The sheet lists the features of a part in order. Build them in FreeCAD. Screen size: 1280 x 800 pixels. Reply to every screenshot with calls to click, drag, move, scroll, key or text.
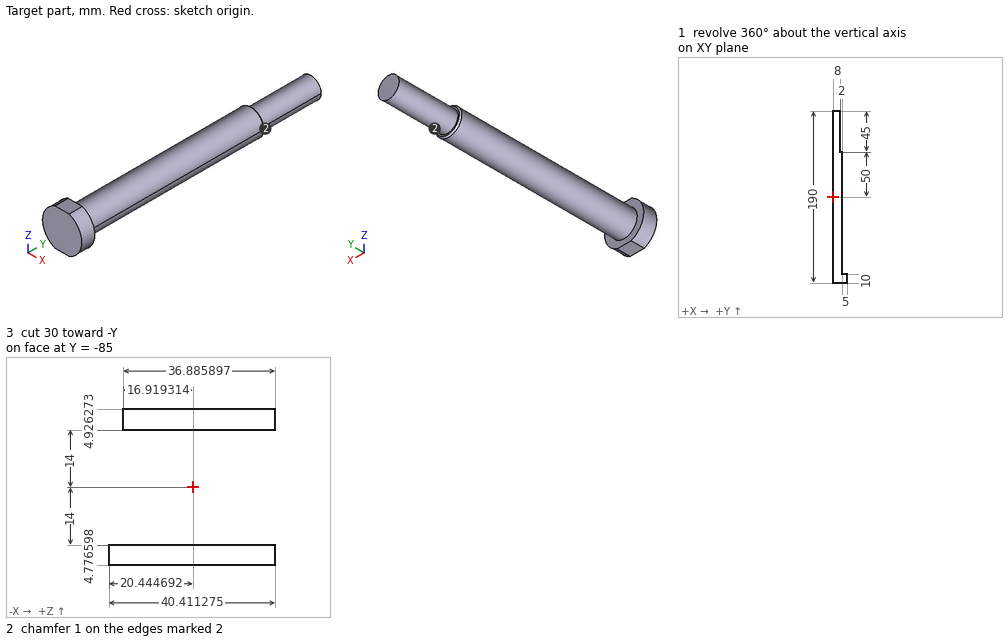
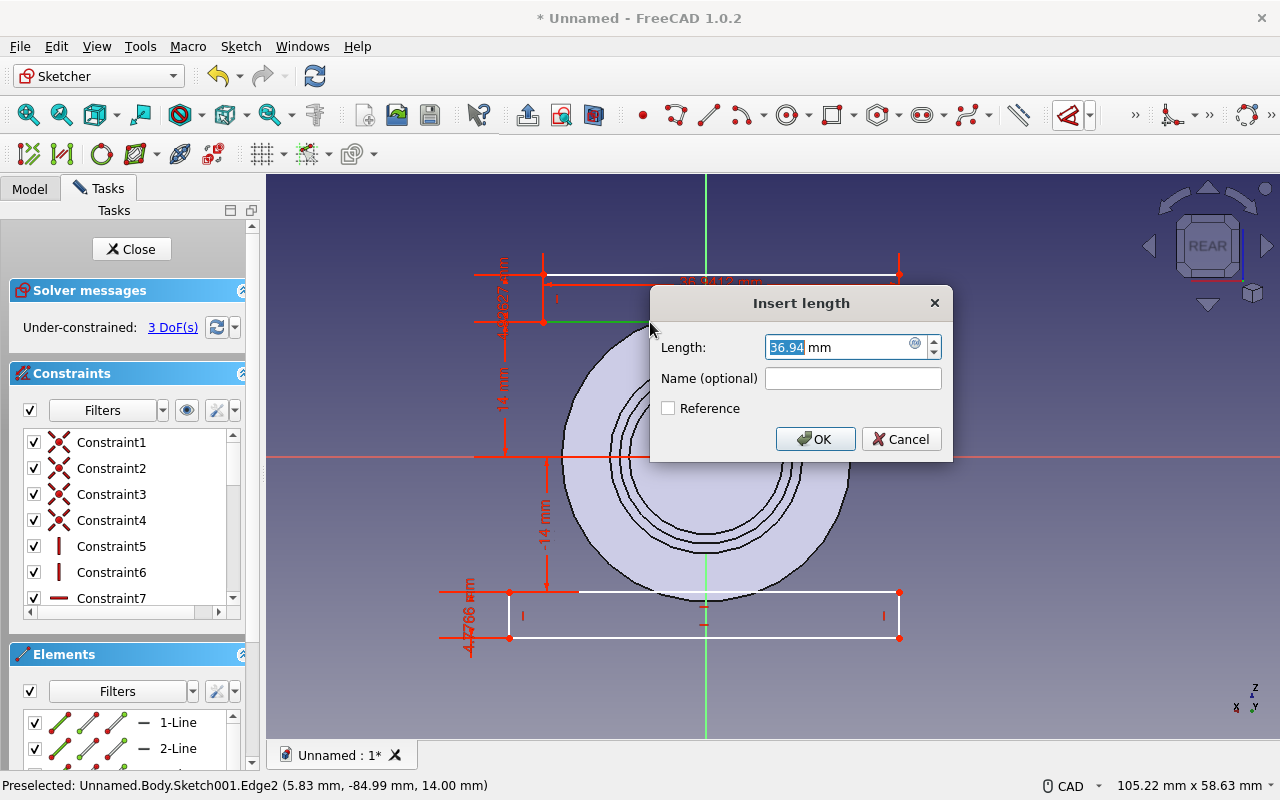
text(36.885897)
key(Return)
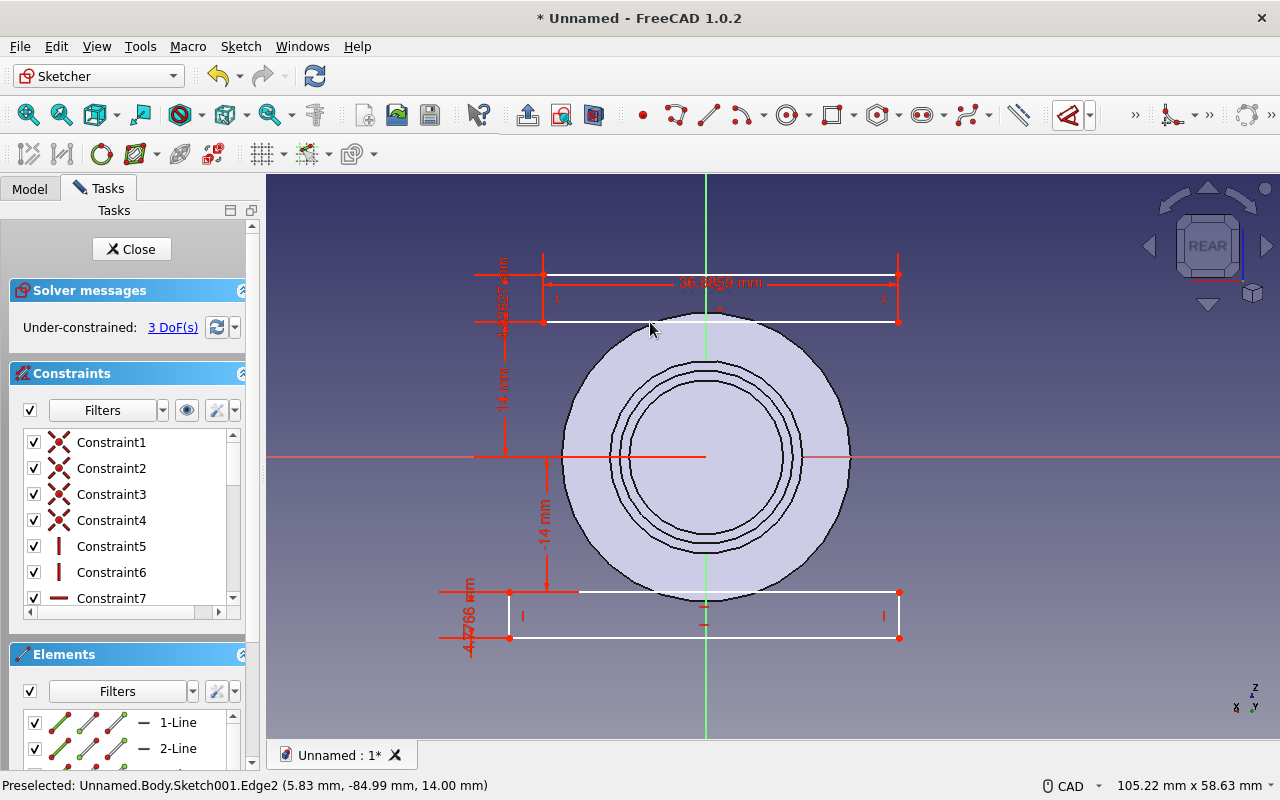
click(626, 638)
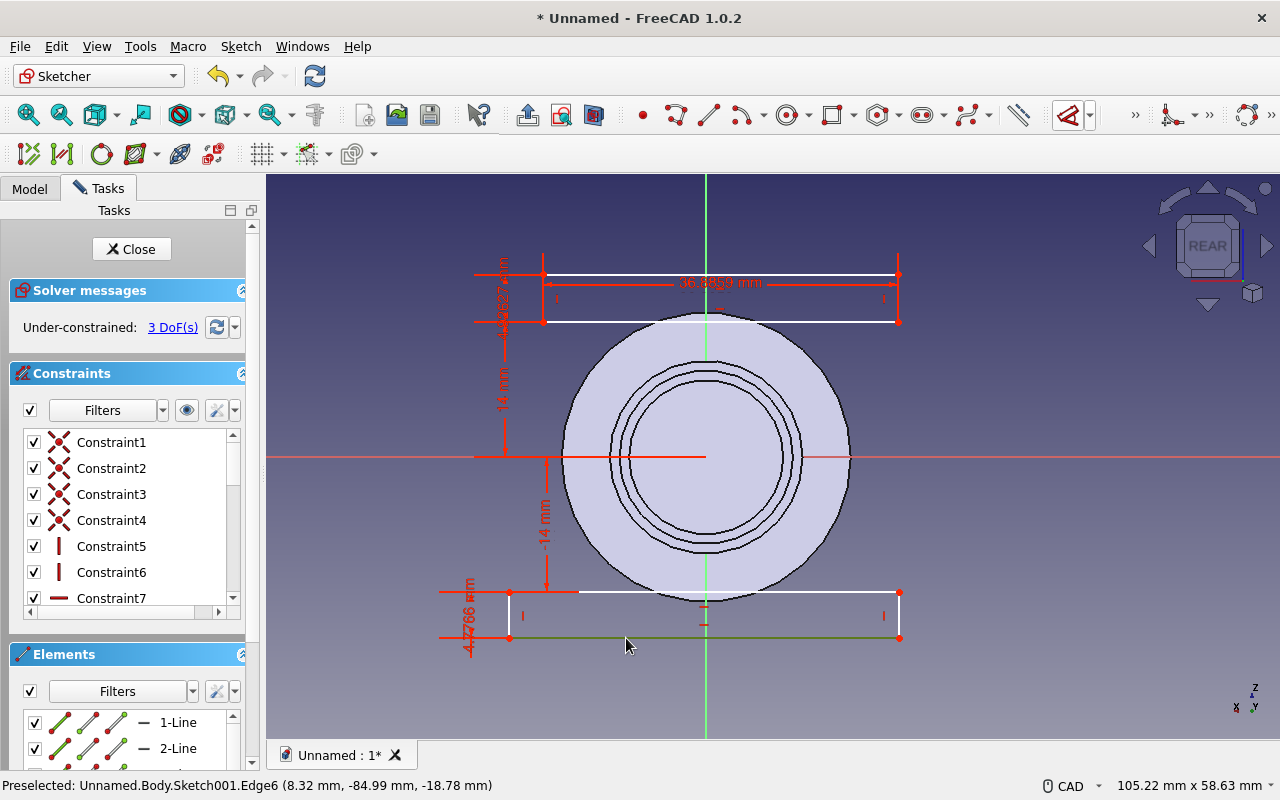
key(l)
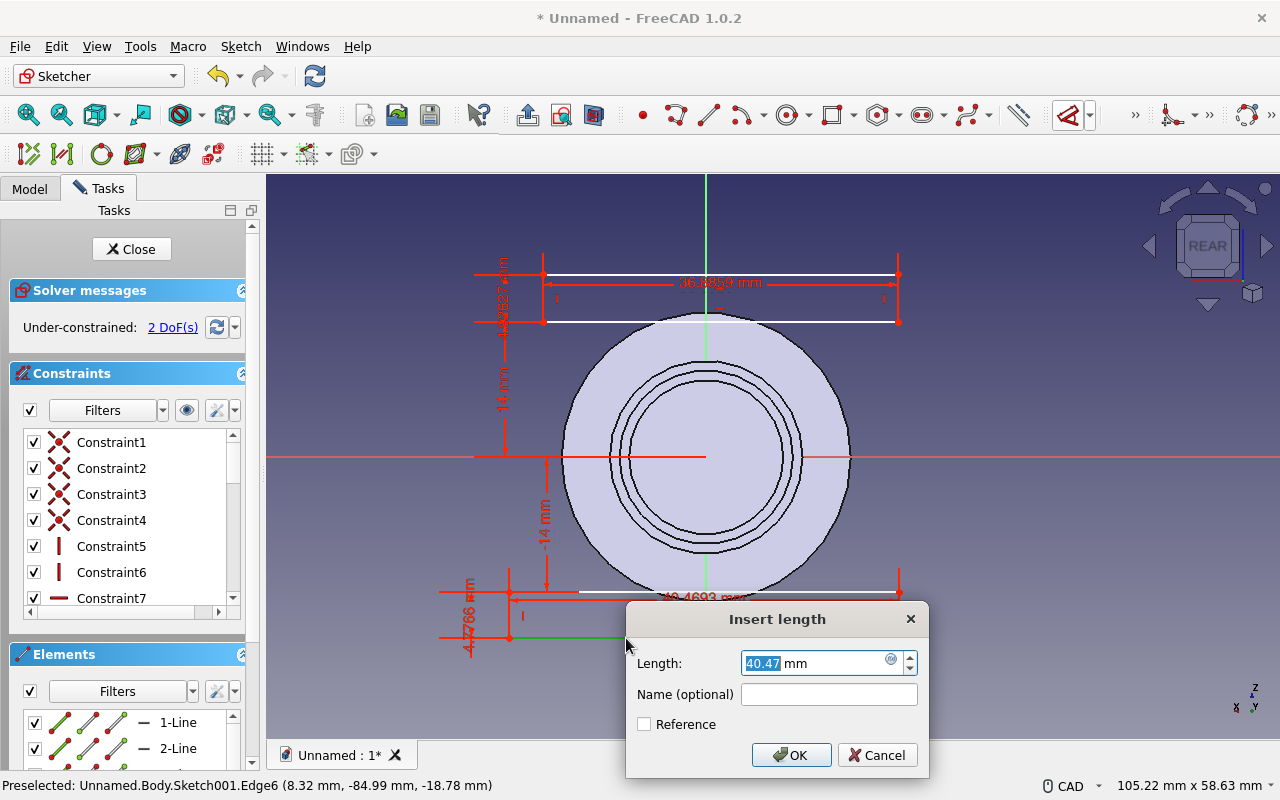
text(40.411275)
key(Return)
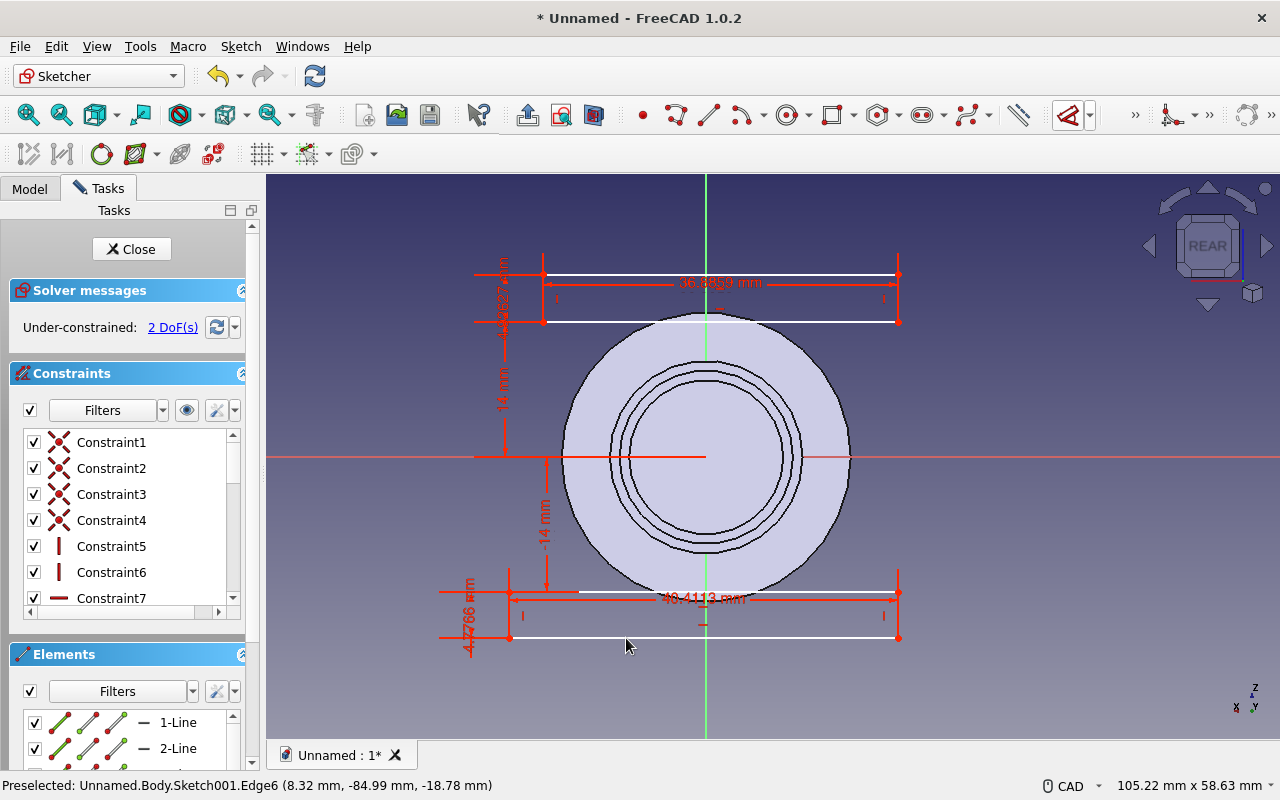
click(543, 275)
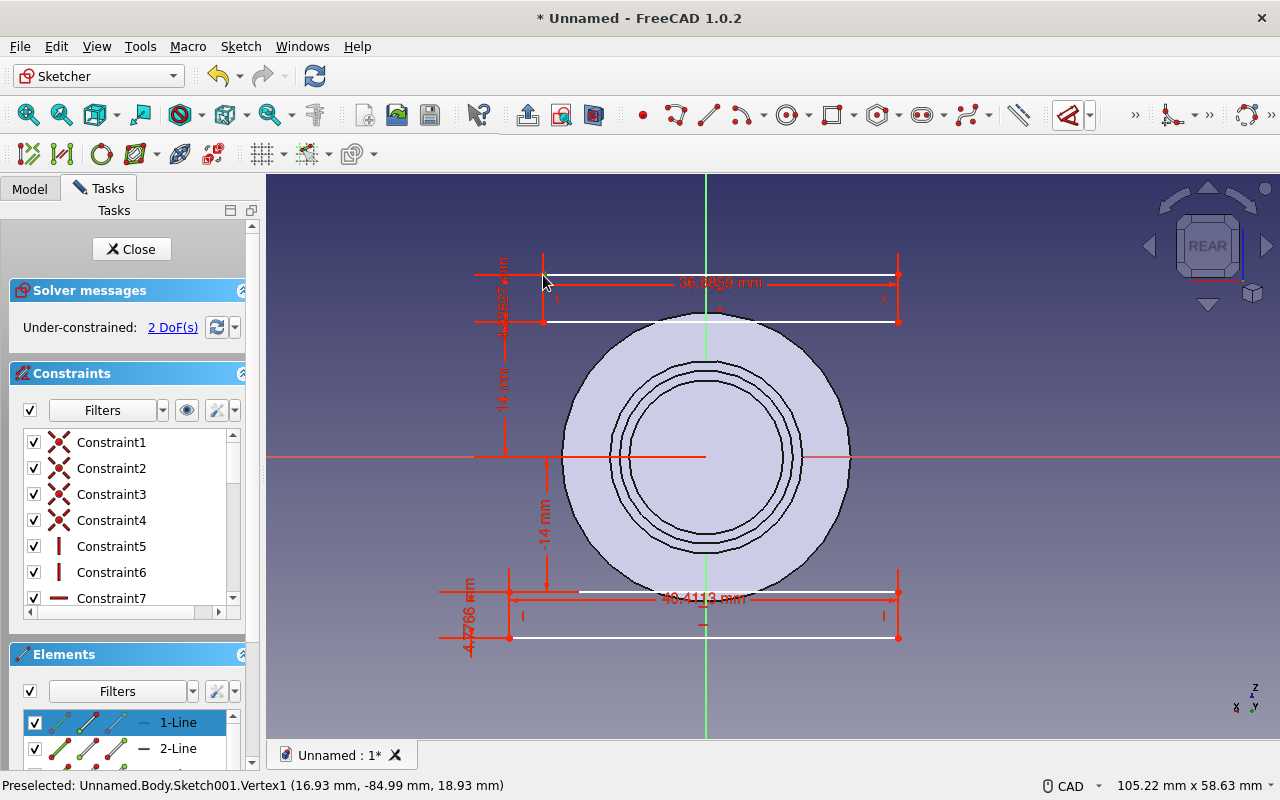
key(l)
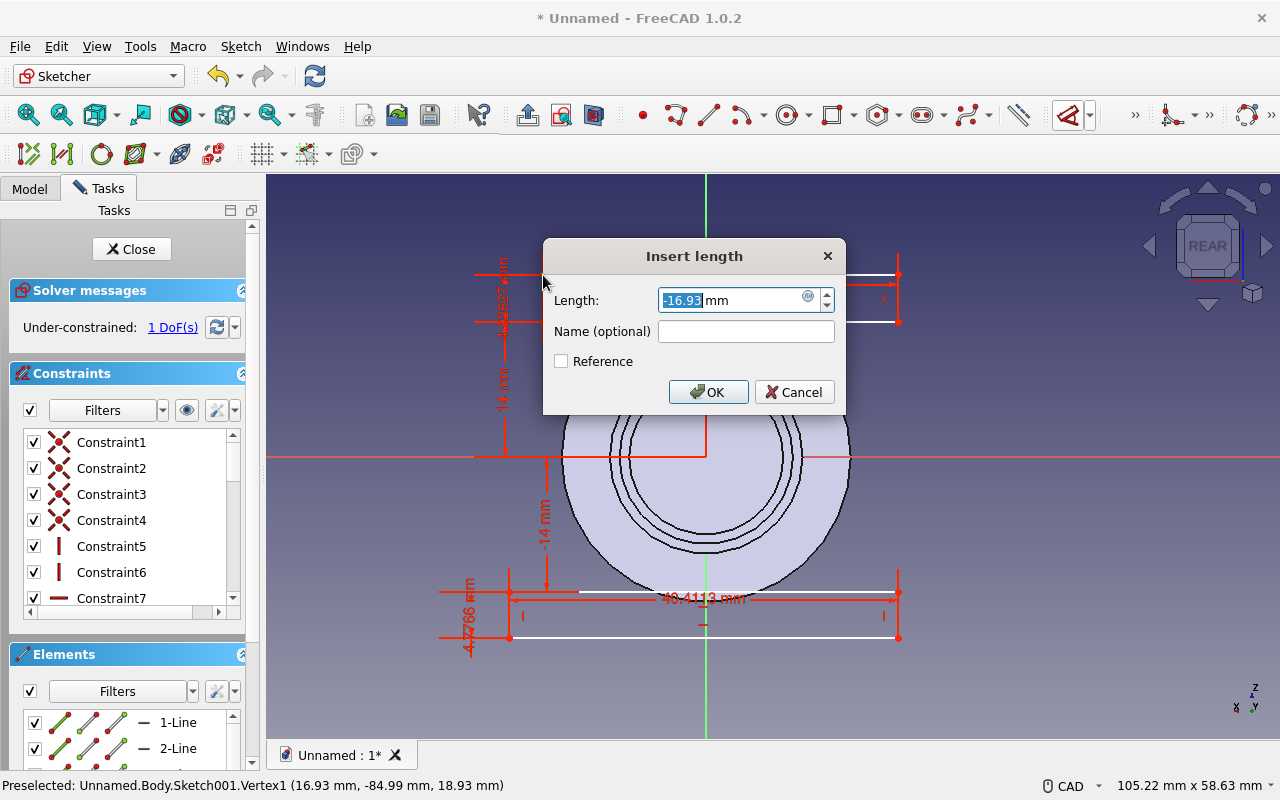
text(-16.919314)
key(Return)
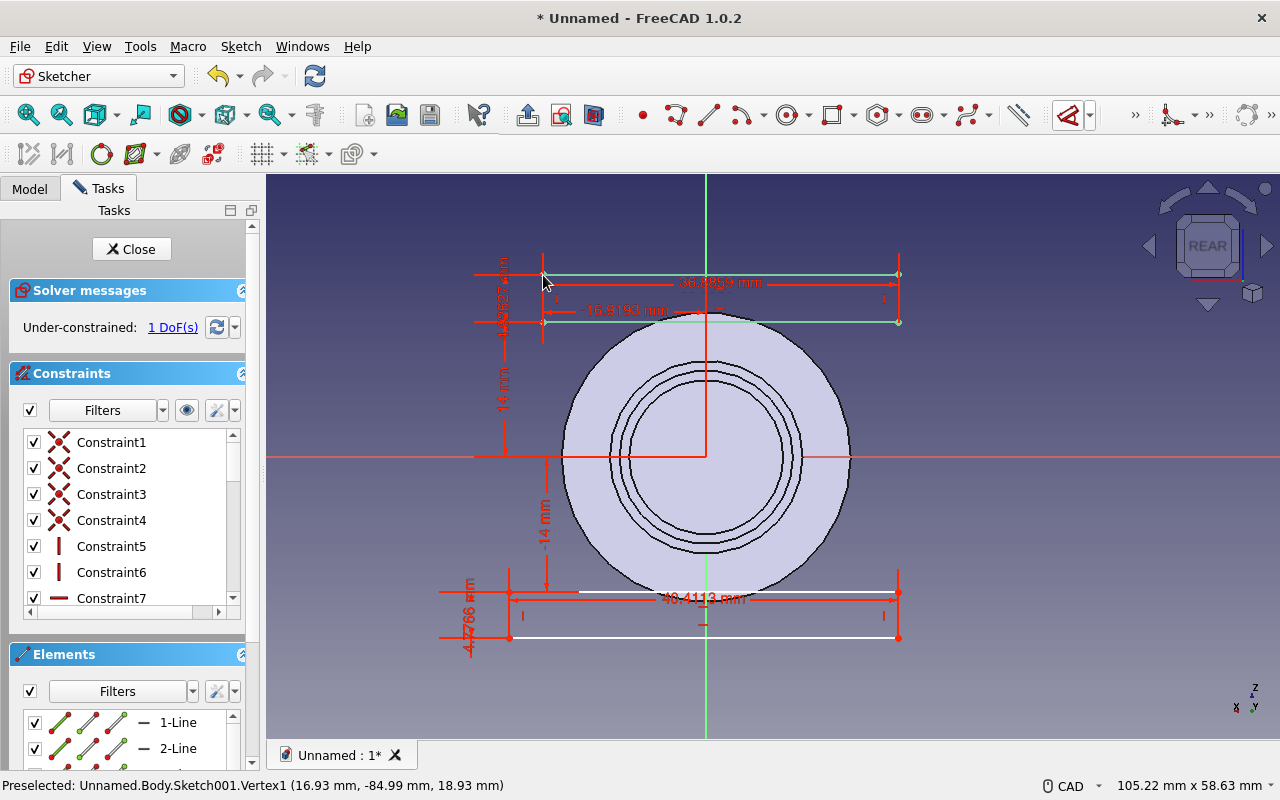
click(509, 592)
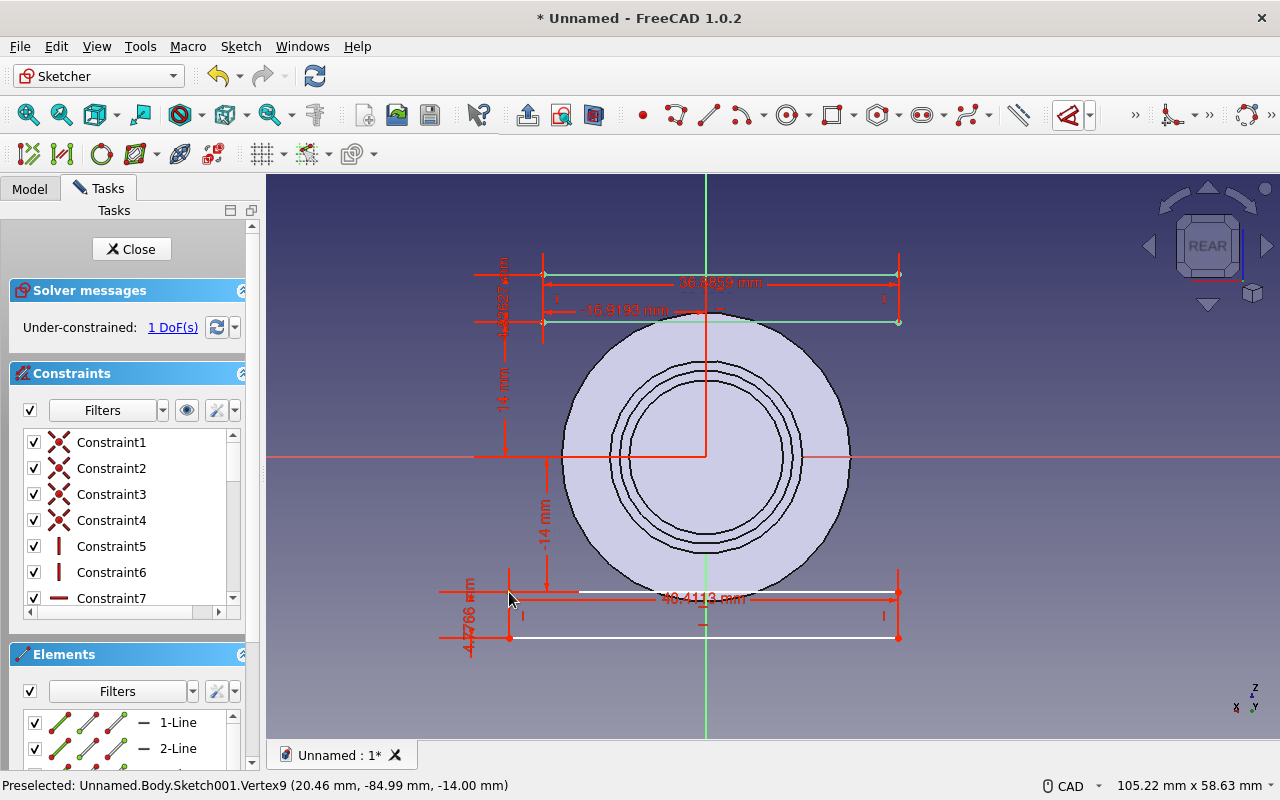
key(l)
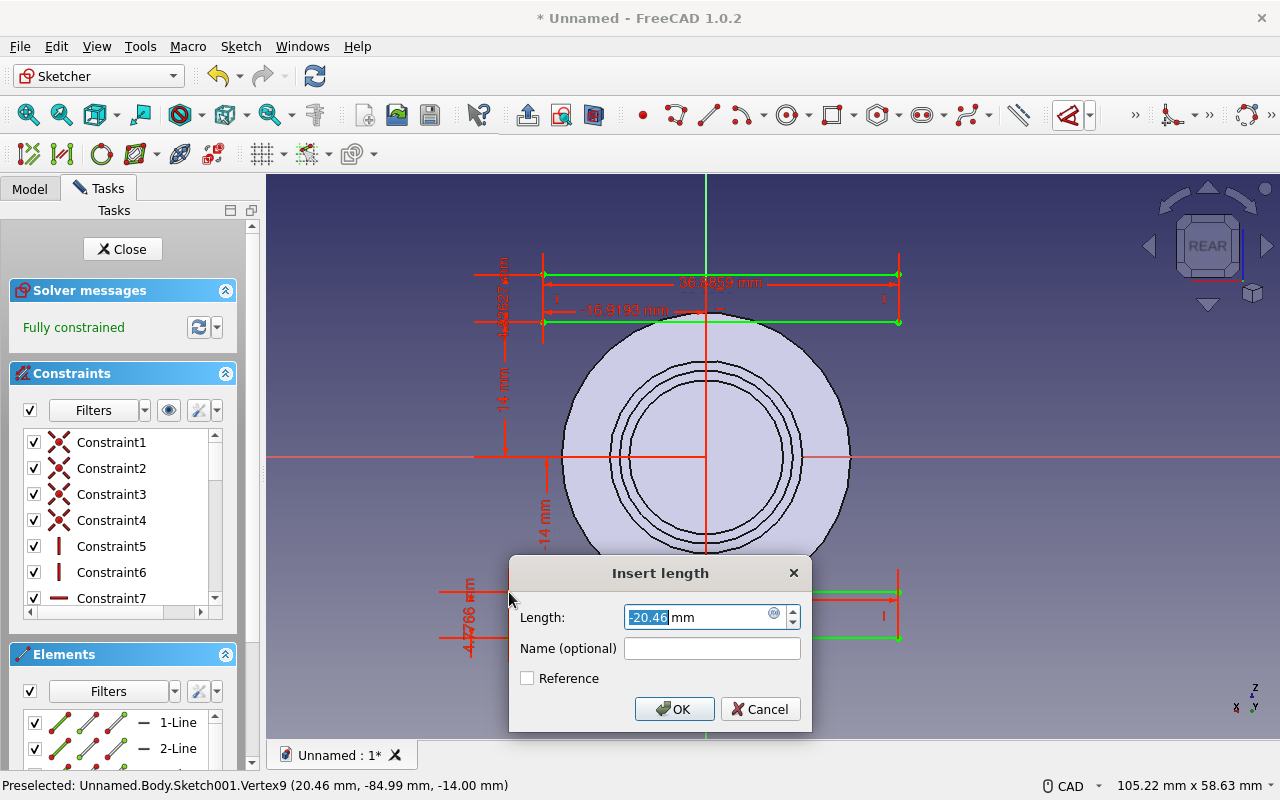
text(-20.444692)
key(Return)